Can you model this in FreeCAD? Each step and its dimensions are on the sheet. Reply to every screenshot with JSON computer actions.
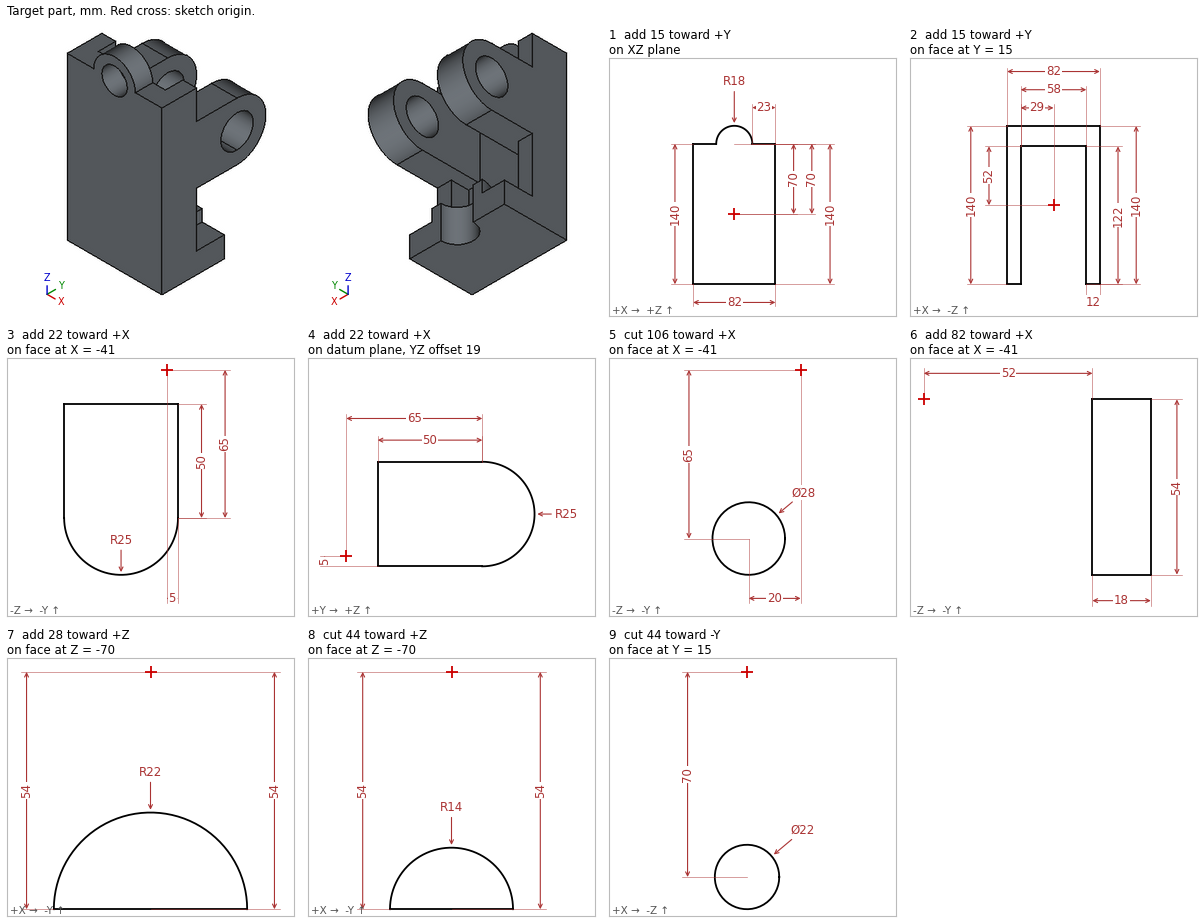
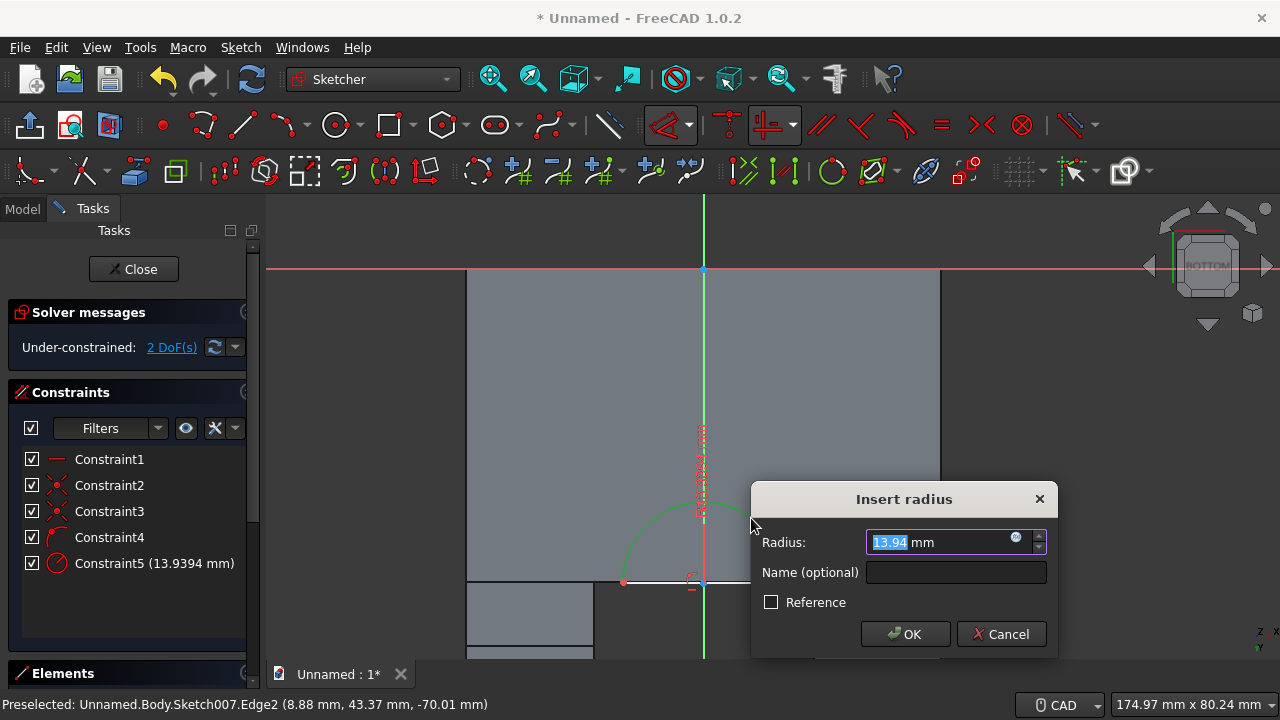
{"action": "type", "text": "14"}
{"action": "key", "text": "Return"}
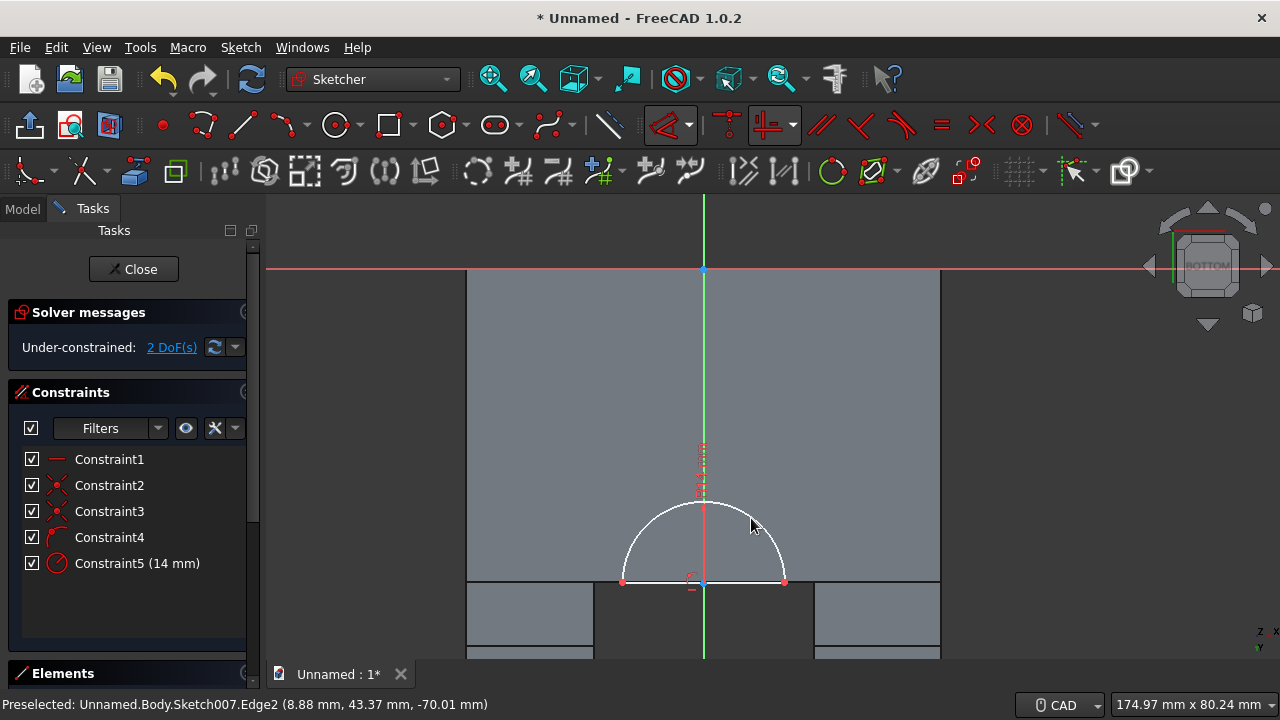
{"action": "left_click", "coordinate": [623, 583]}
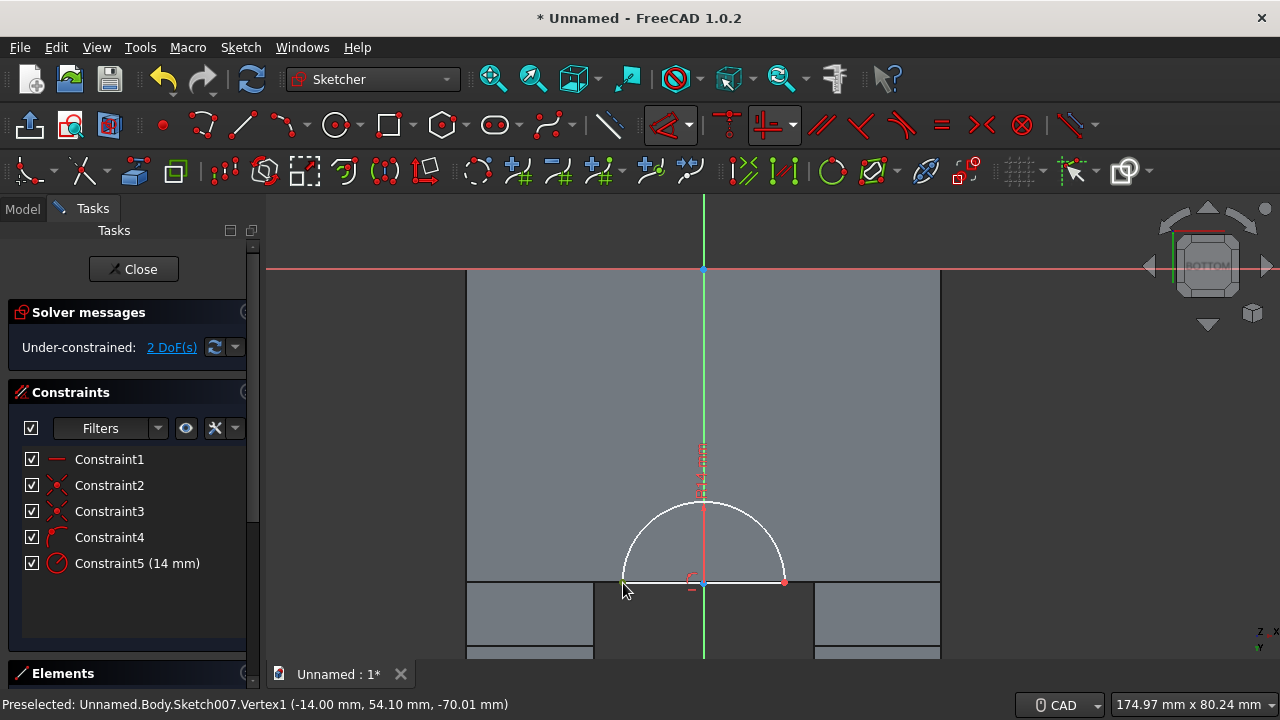
{"action": "key", "text": "i"}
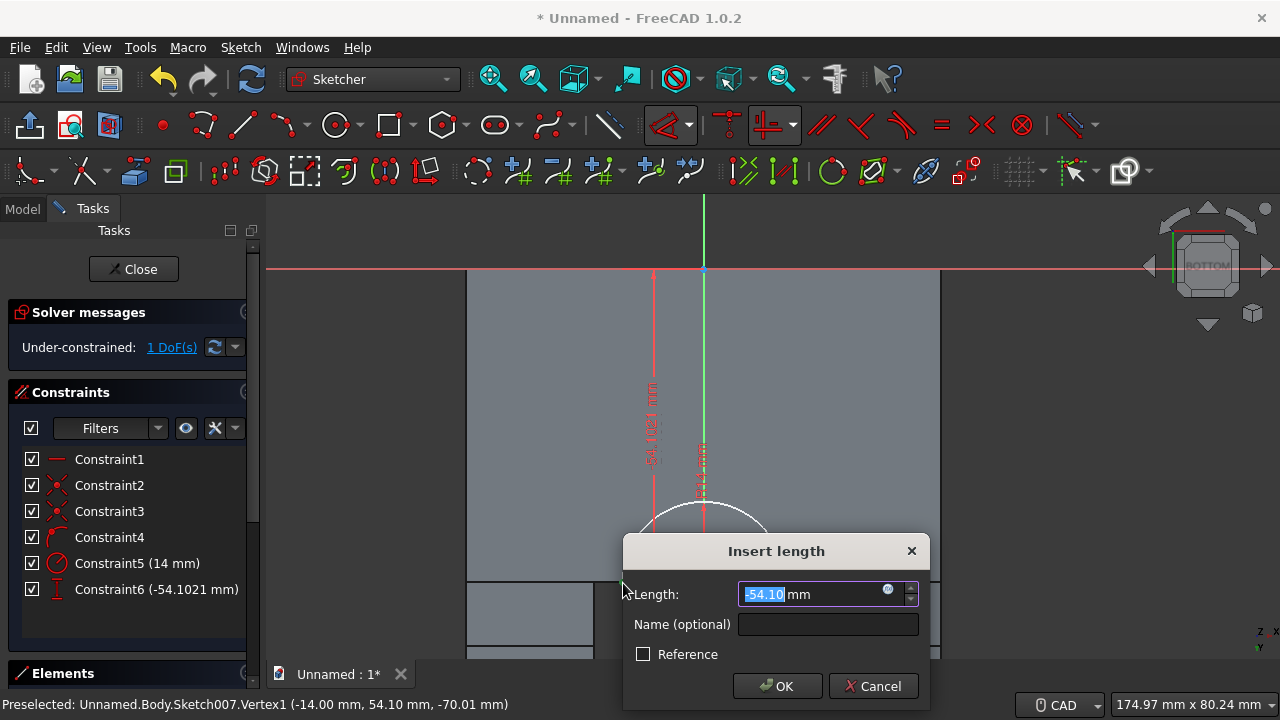
{"action": "type", "text": "-54"}
{"action": "key", "text": "Return"}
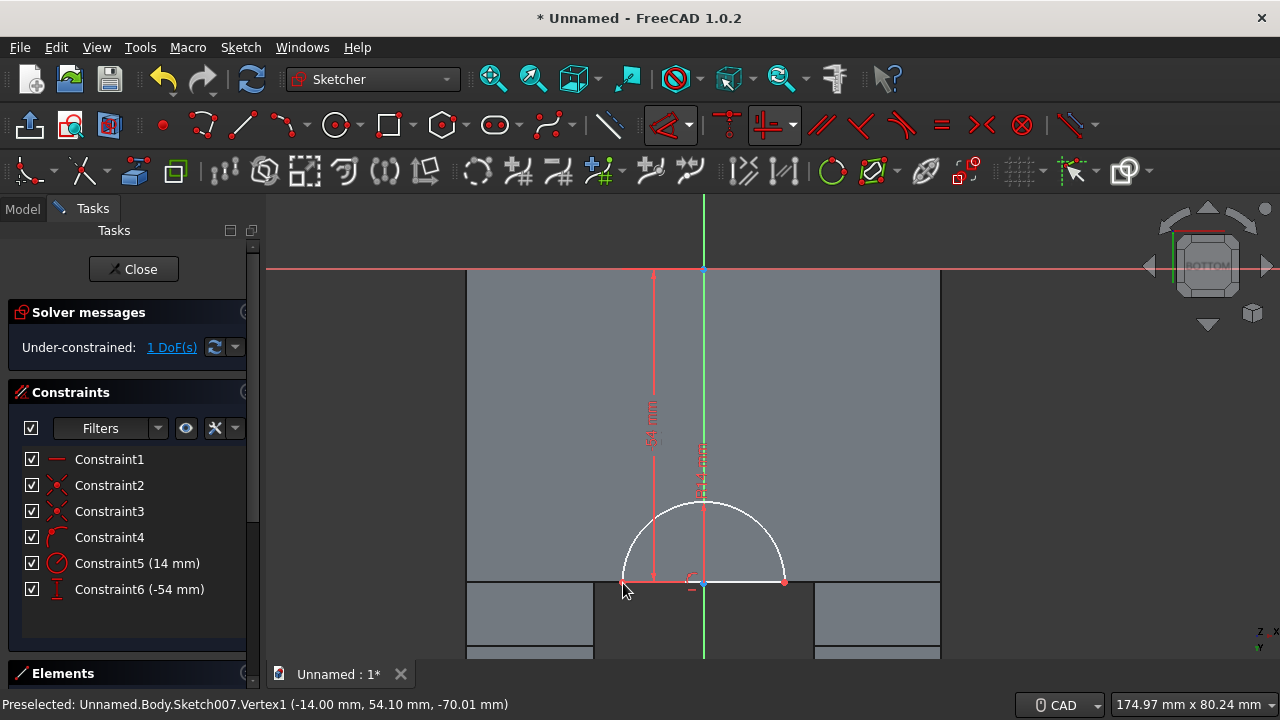
{"action": "left_click", "coordinate": [704, 583]}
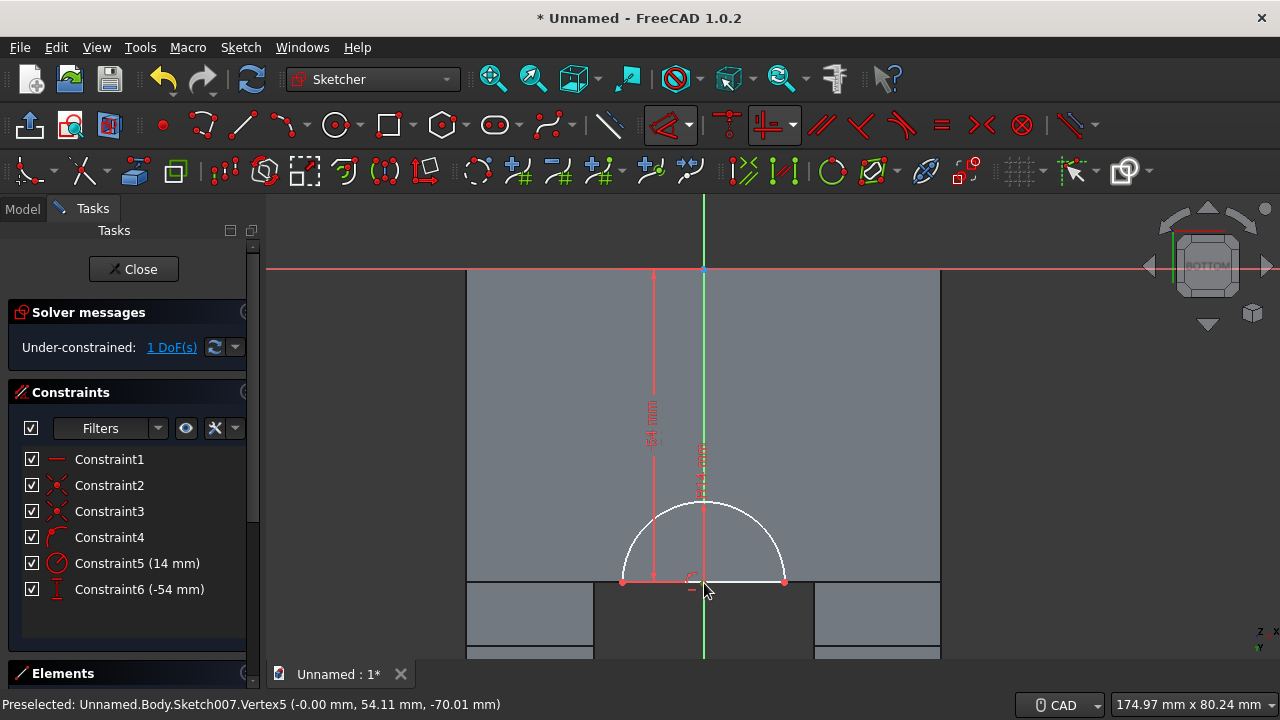
{"action": "key", "text": "i"}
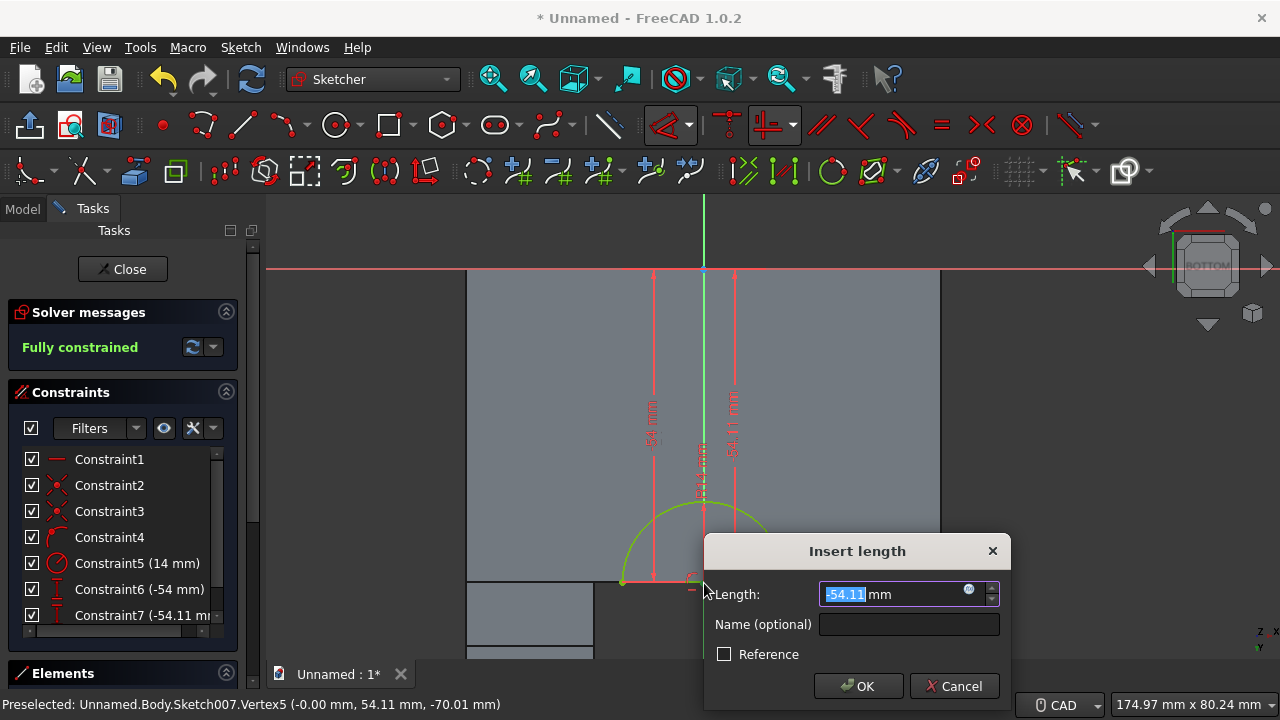
{"action": "type", "text": "-54"}
{"action": "key", "text": "Return"}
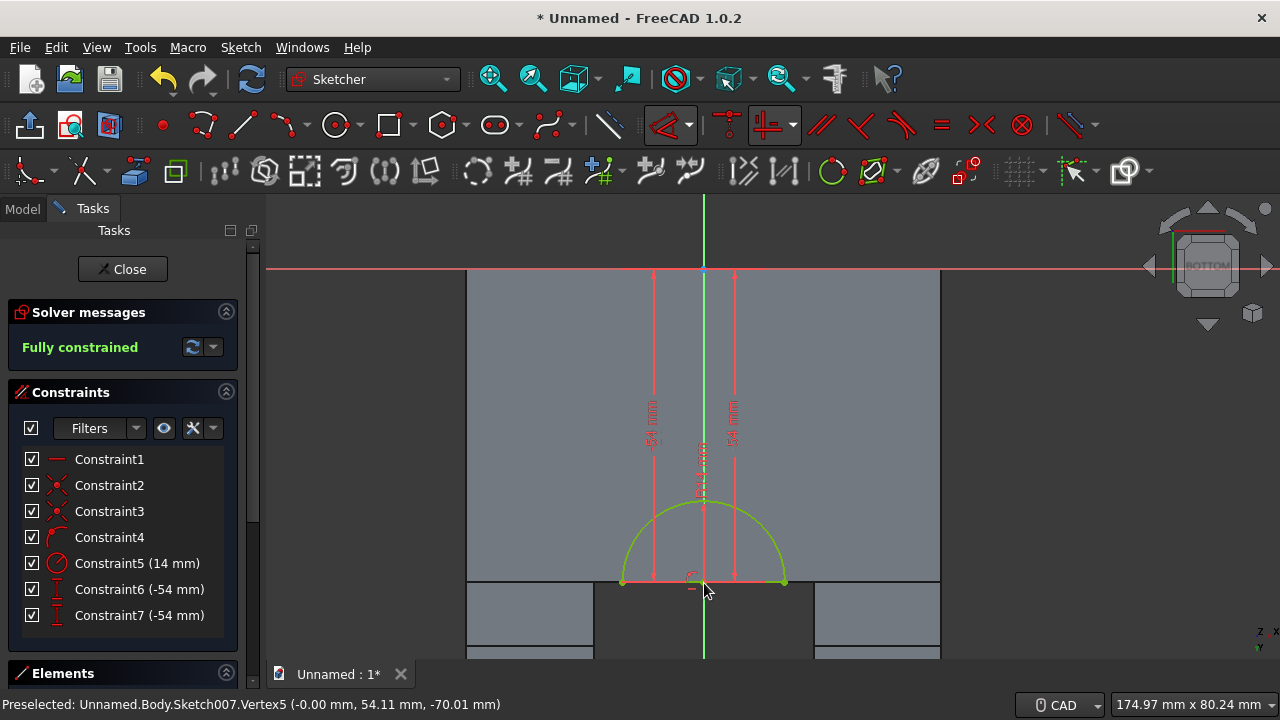
{"action": "left_click", "coordinate": [123, 269]}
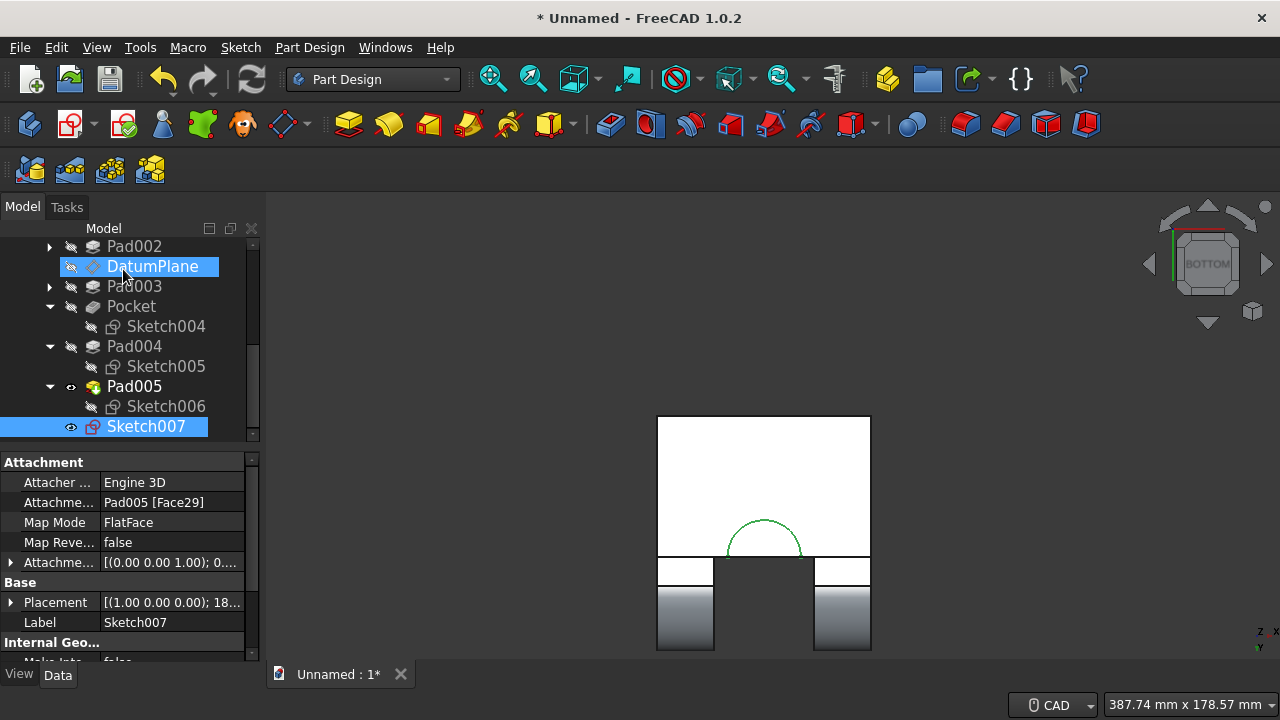
{"action": "left_click", "coordinate": [612, 124]}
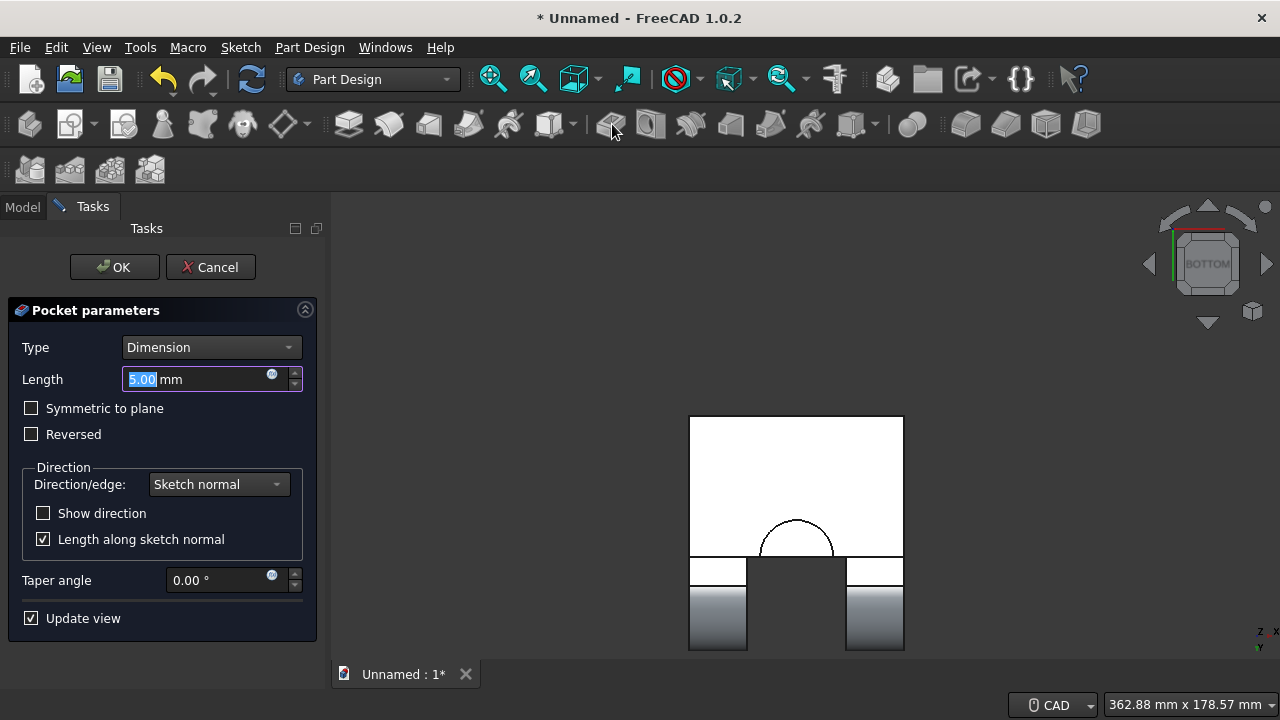
{"action": "type", "text": "44"}
{"action": "key", "text": "Tab"}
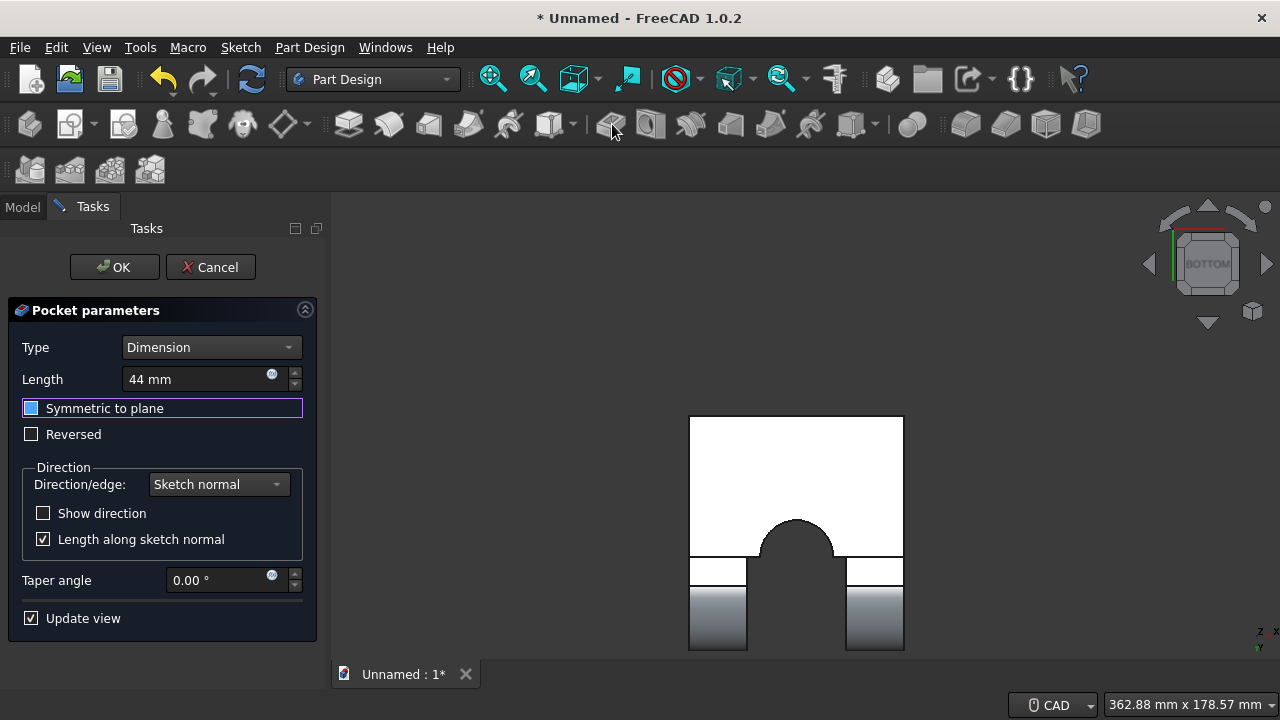
{"action": "left_click", "coordinate": [115, 267]}